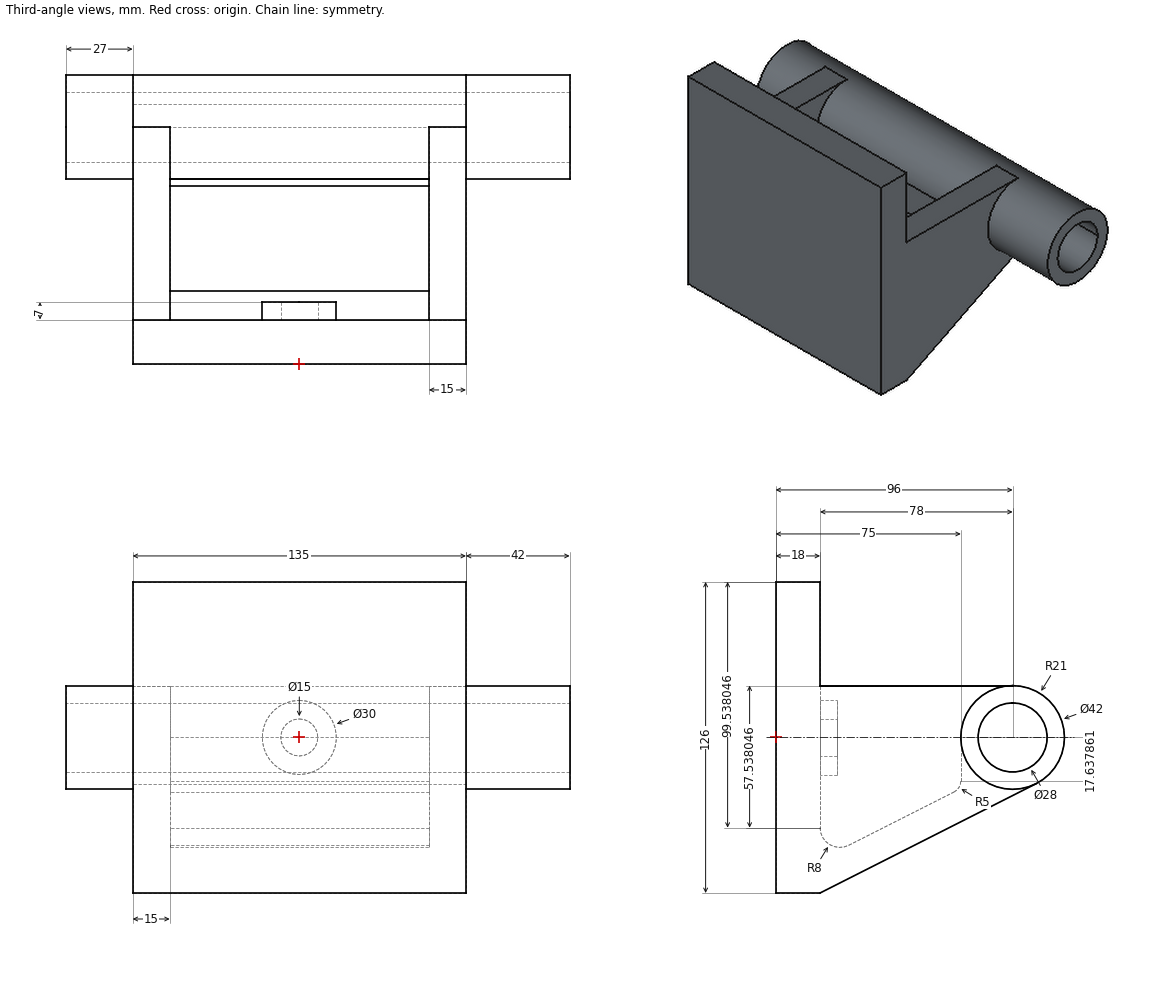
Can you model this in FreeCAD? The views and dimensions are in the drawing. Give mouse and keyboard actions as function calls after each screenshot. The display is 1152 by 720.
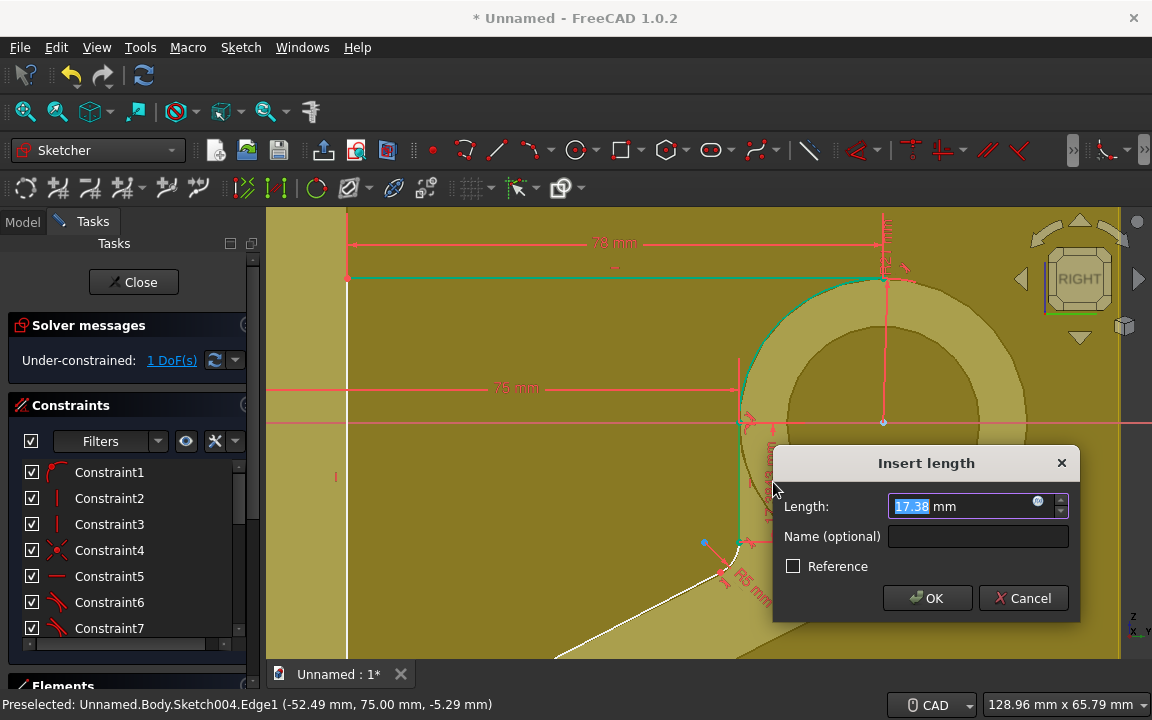
text(17.637861)
key(Return)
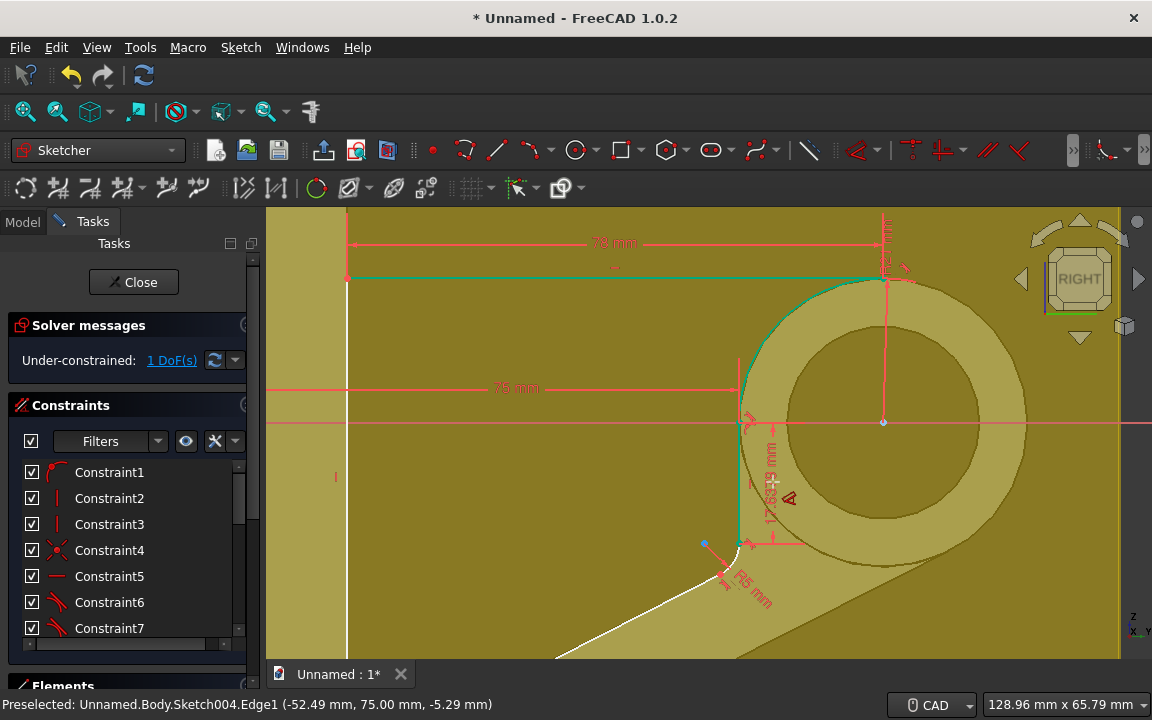
click(347, 556)
click(313, 455)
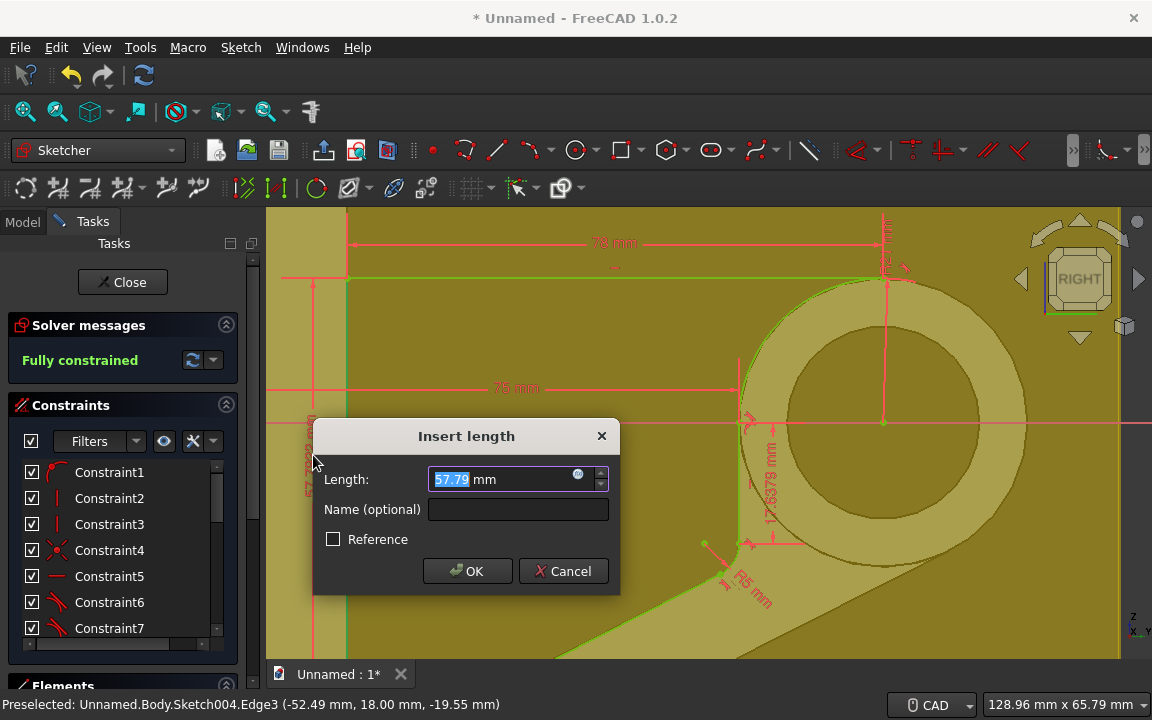
text(57.538046)
key(Return)
key(Escape)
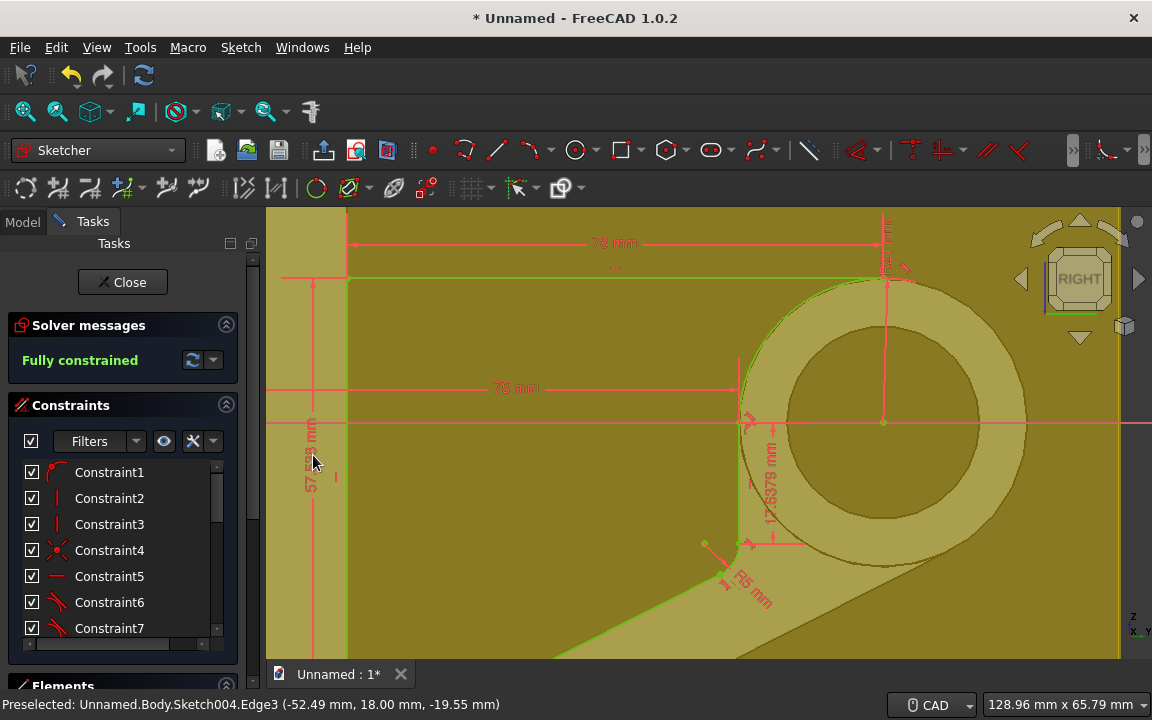
click(123, 282)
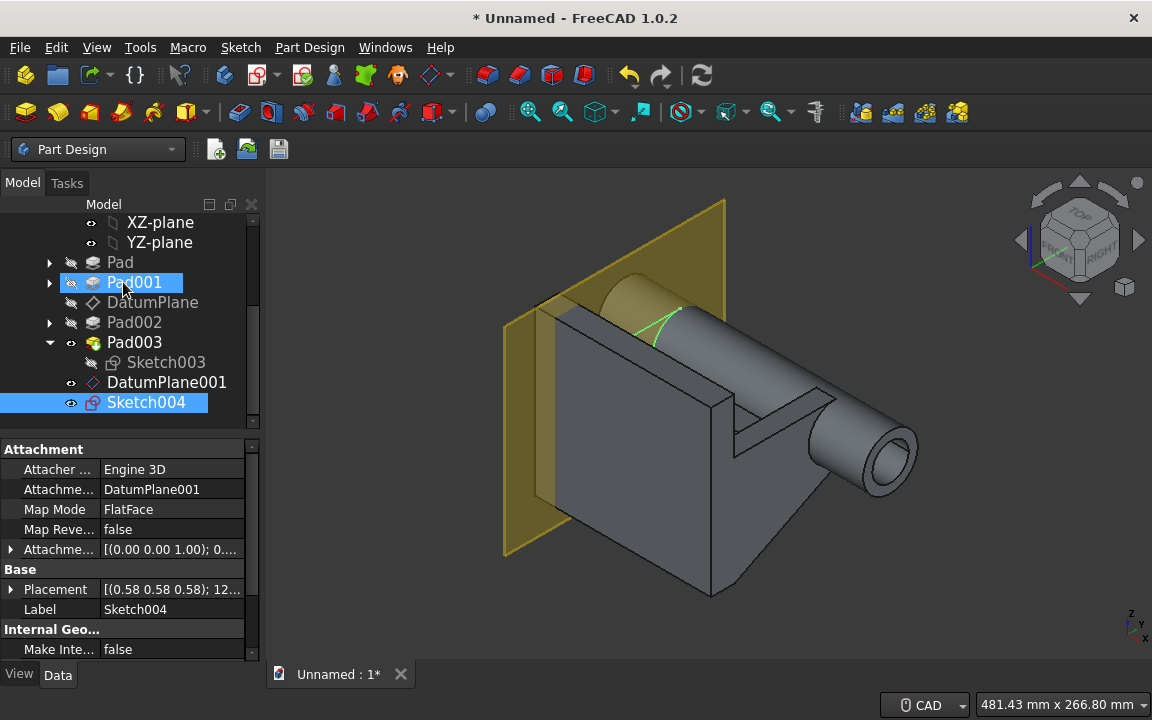
click(26, 112)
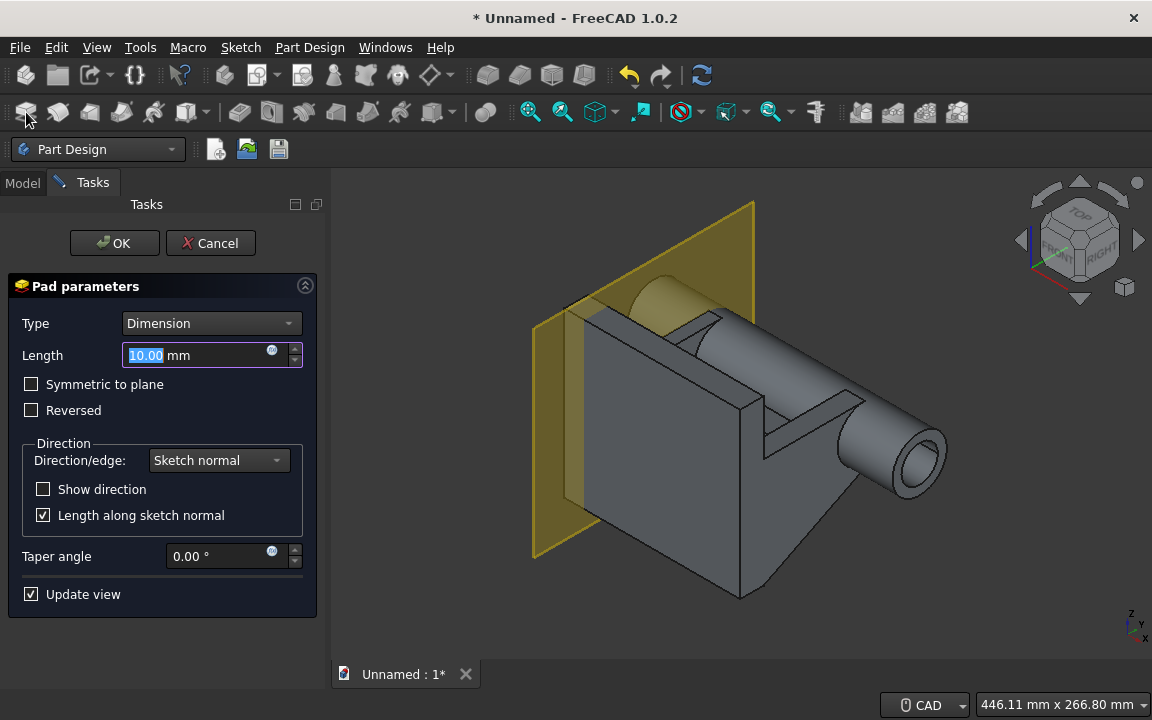
text(15)
key(Tab)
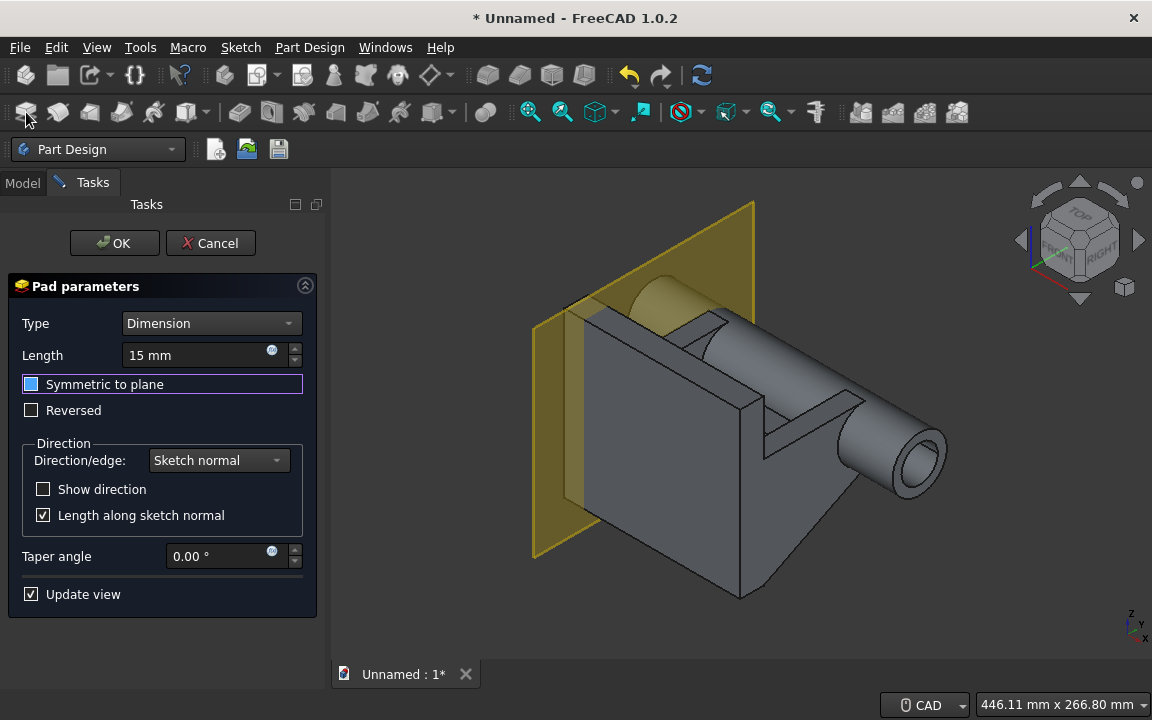
click(30, 410)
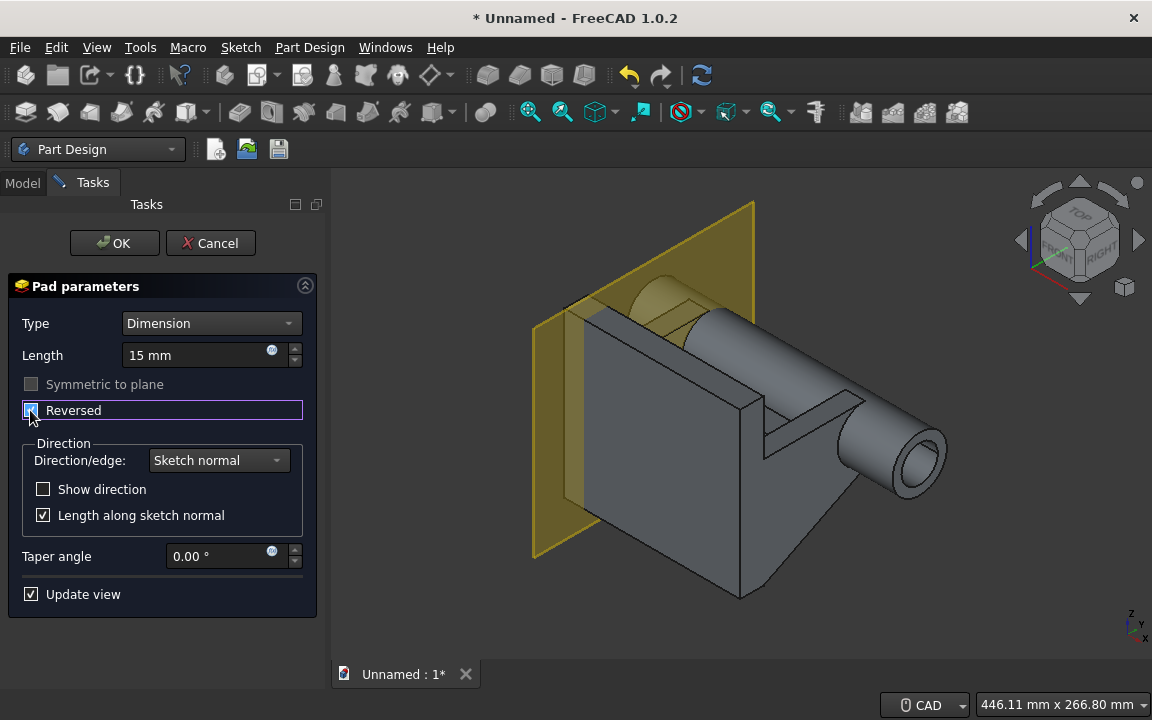
click(115, 243)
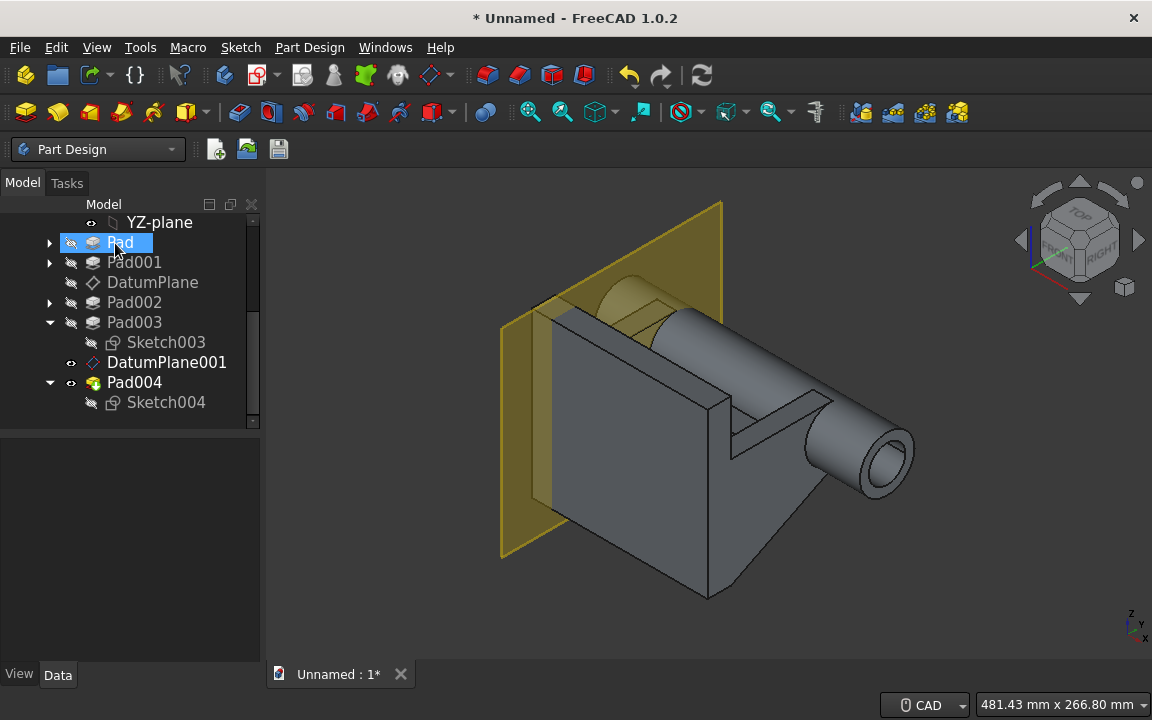
click(116, 363)
key(space)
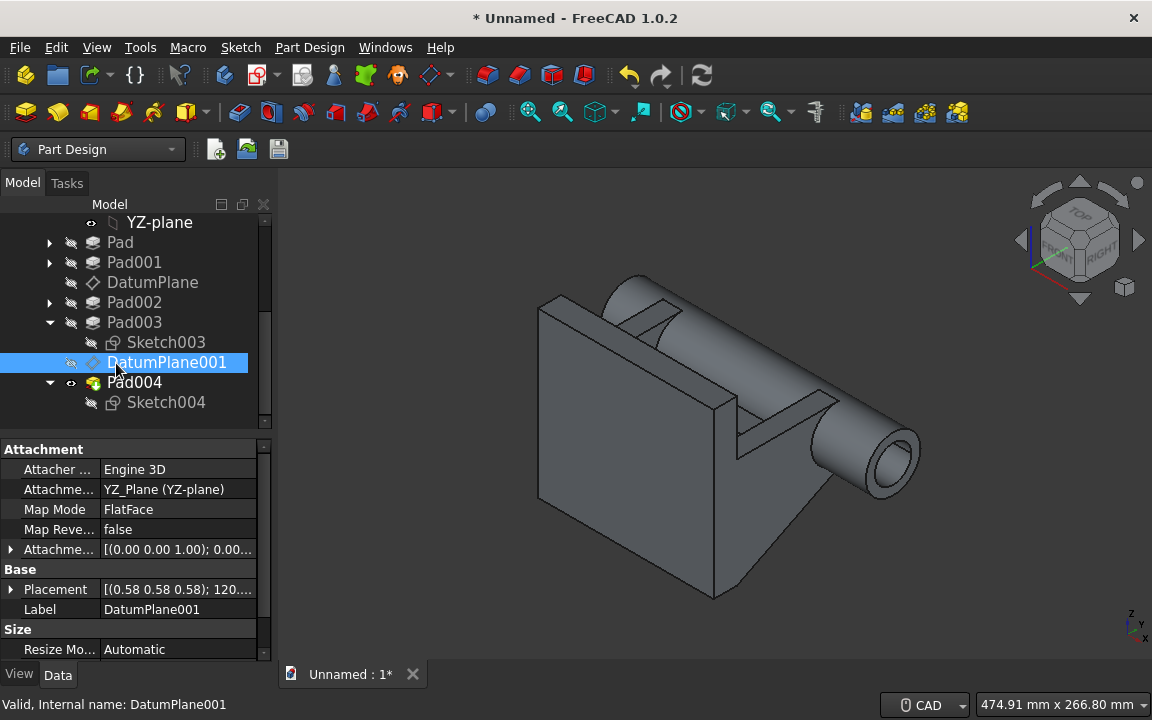
key(4)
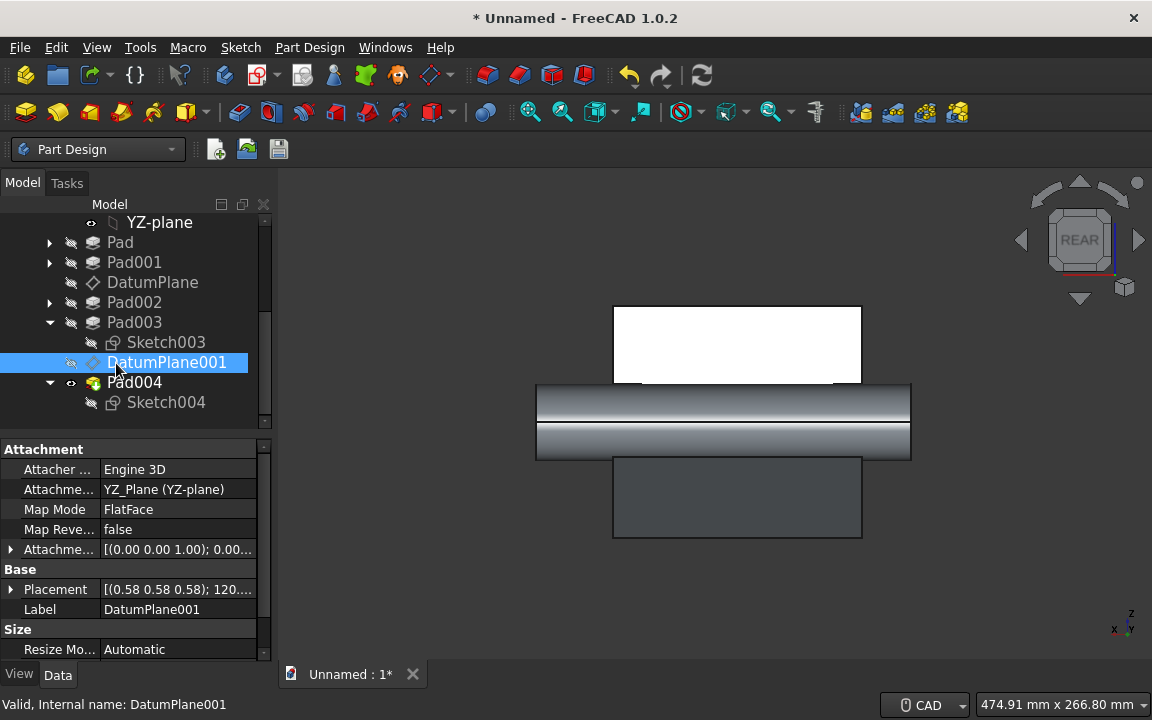
click(738, 371)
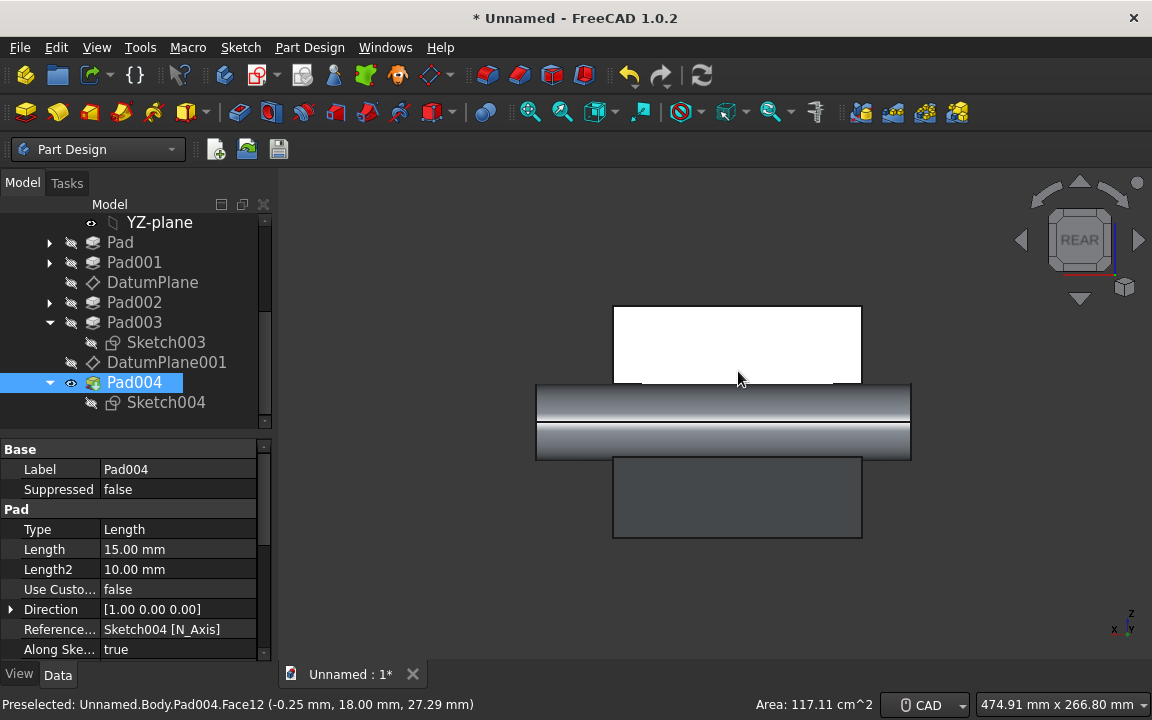
click(258, 76)